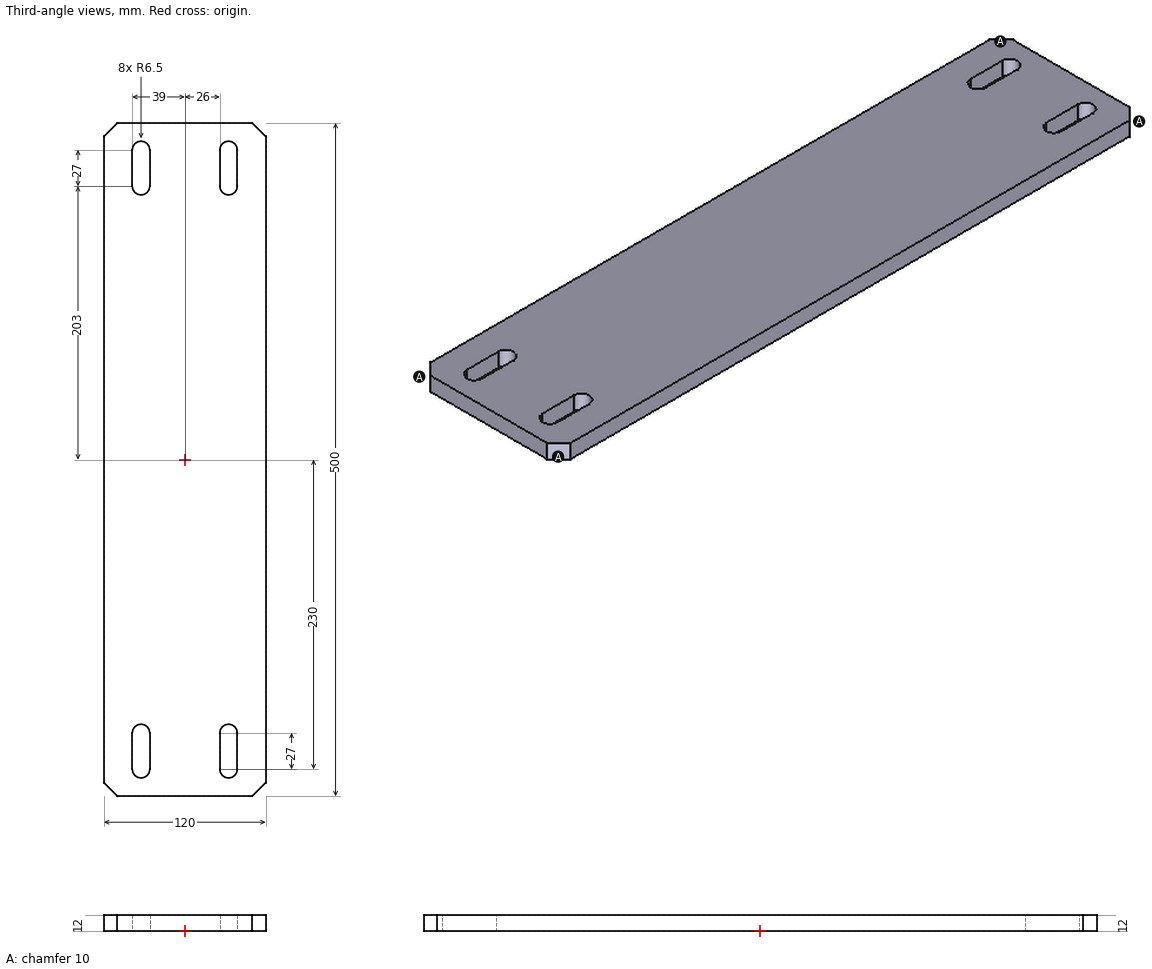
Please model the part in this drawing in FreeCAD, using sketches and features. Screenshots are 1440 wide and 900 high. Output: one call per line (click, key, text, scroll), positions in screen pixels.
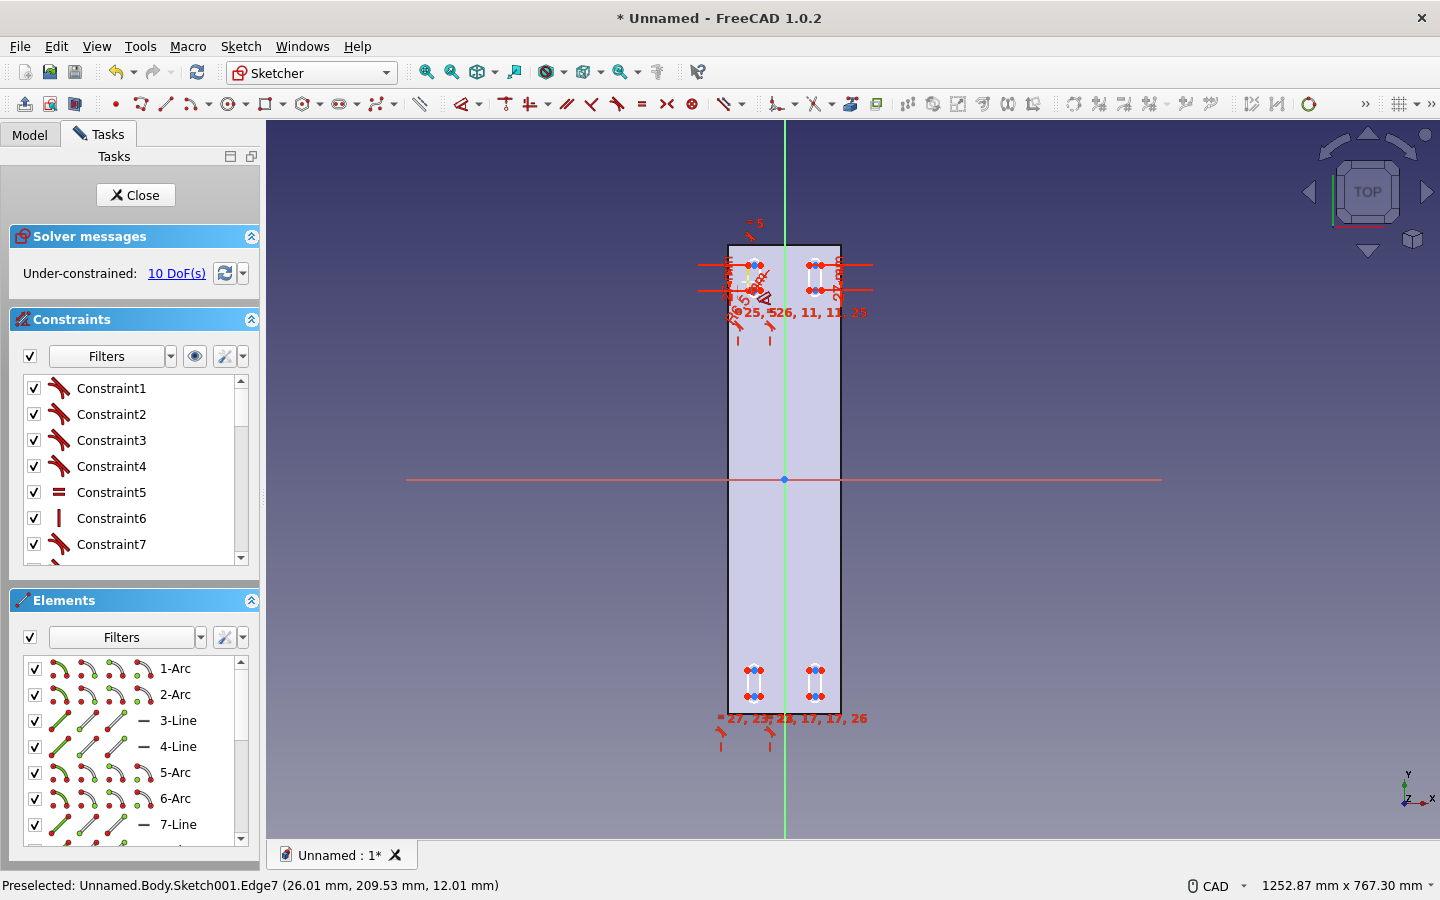
scroll(809, 689, up, 3)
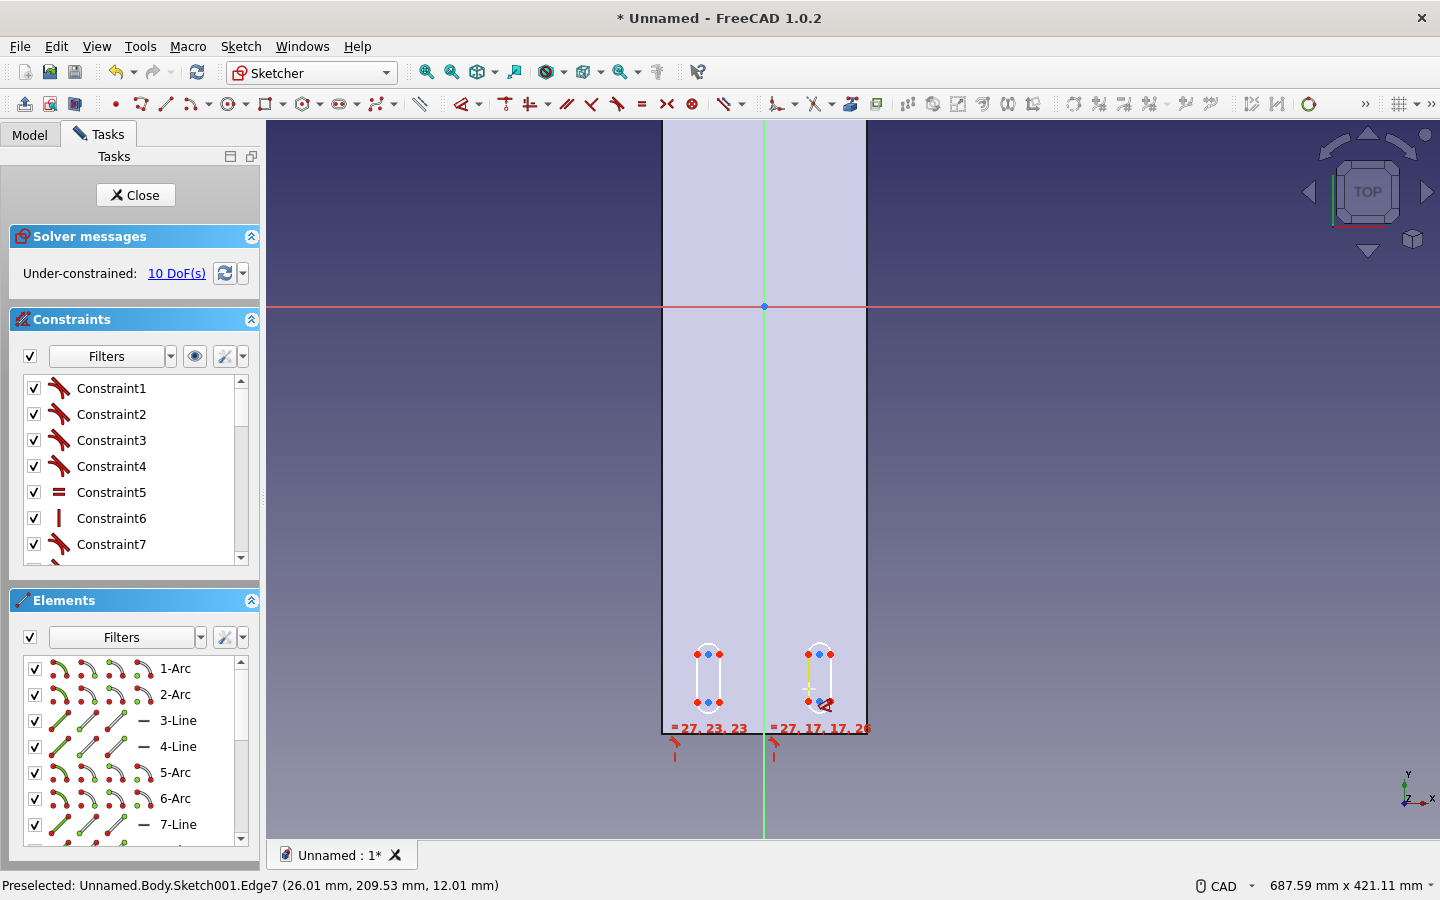
click(809, 687)
click(867, 678)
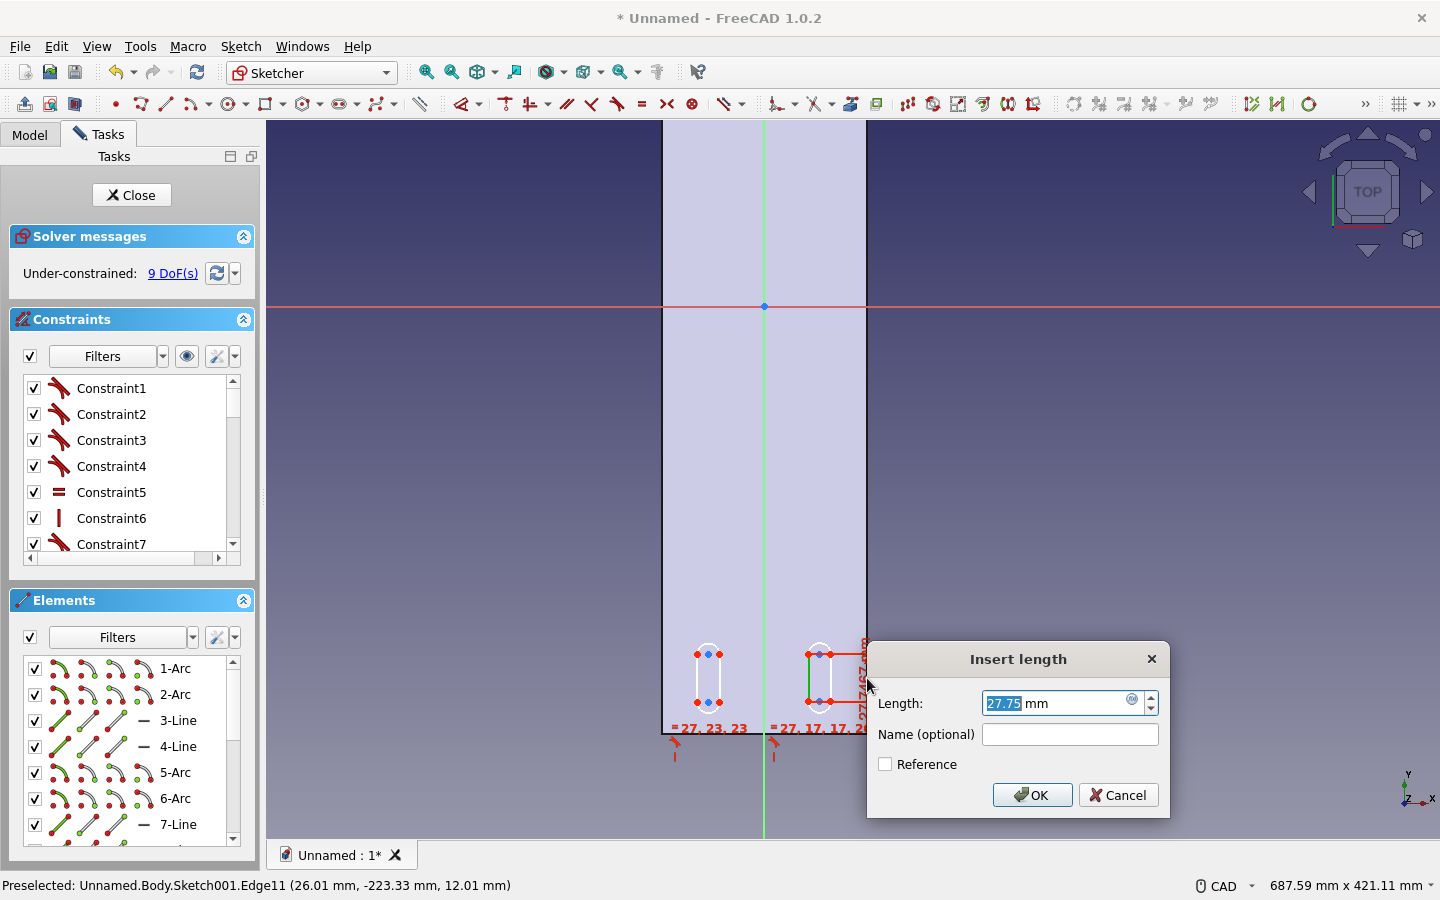
text(27)
key(Return)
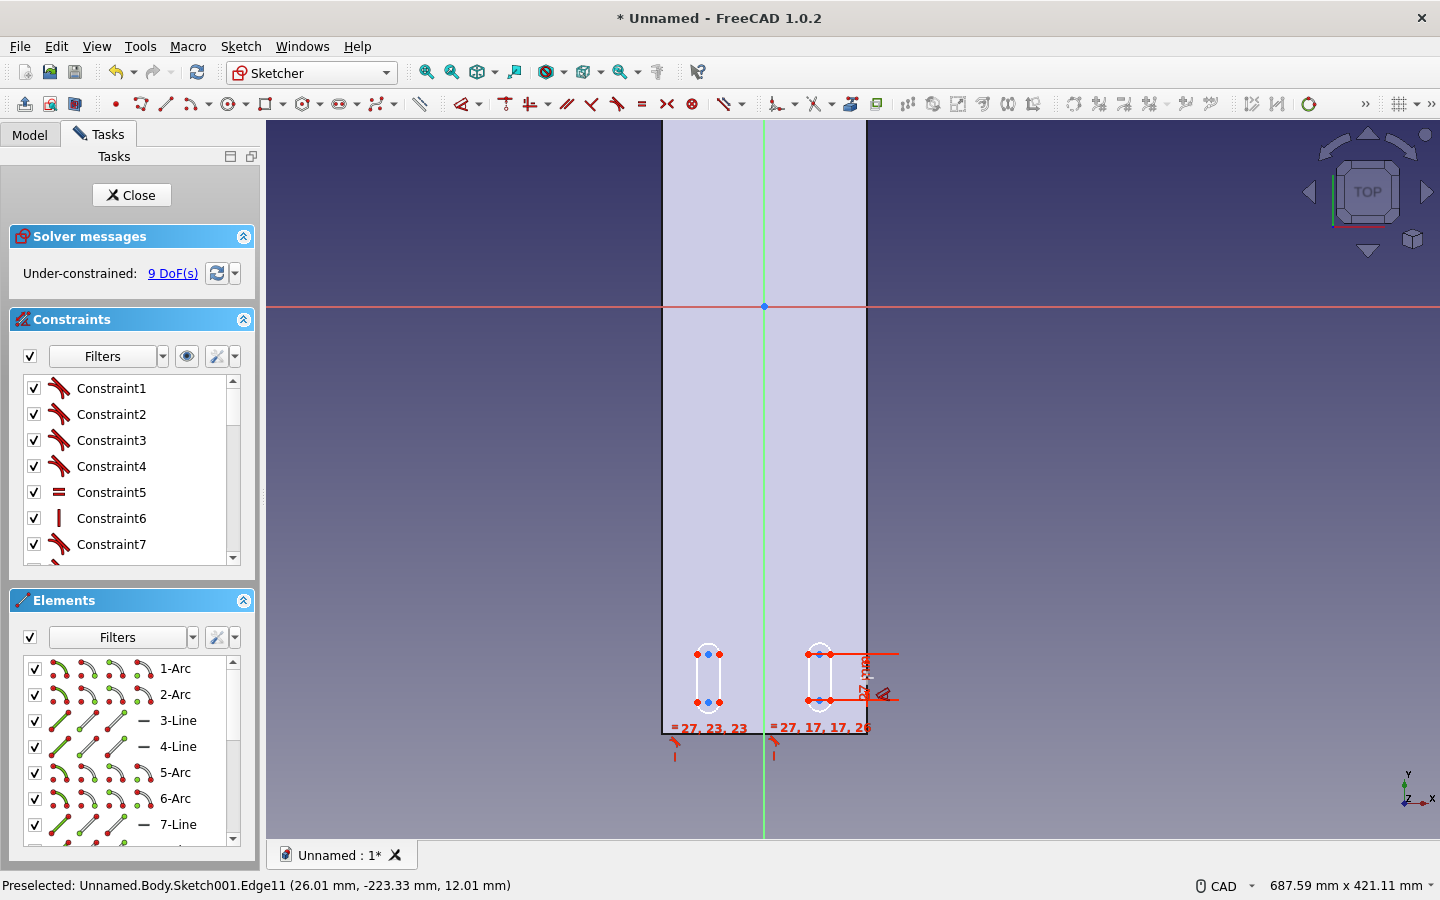
click(697, 688)
click(663, 678)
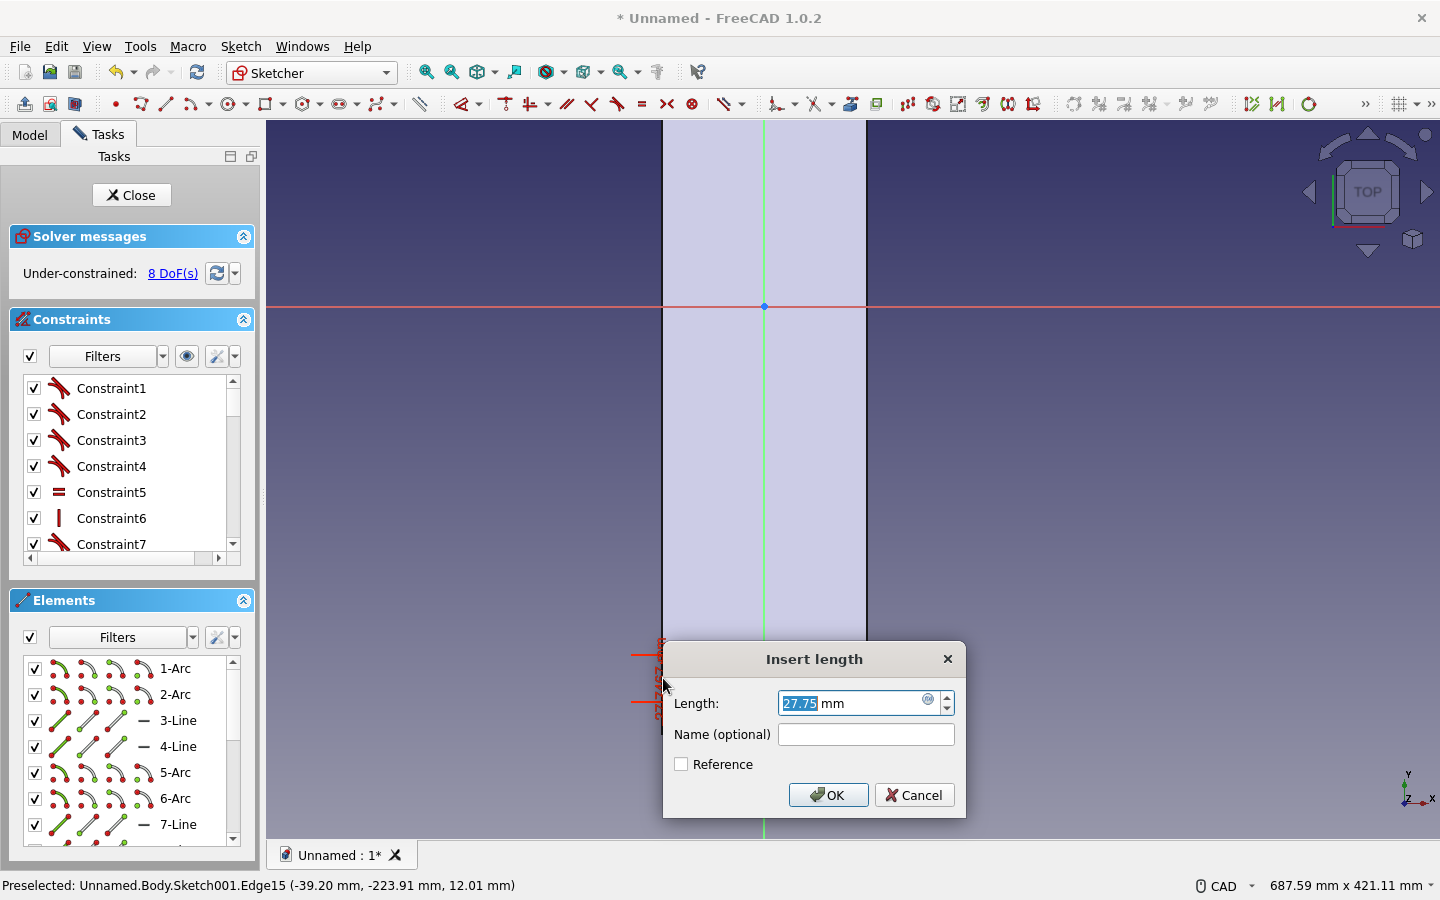
text(27)
key(Return)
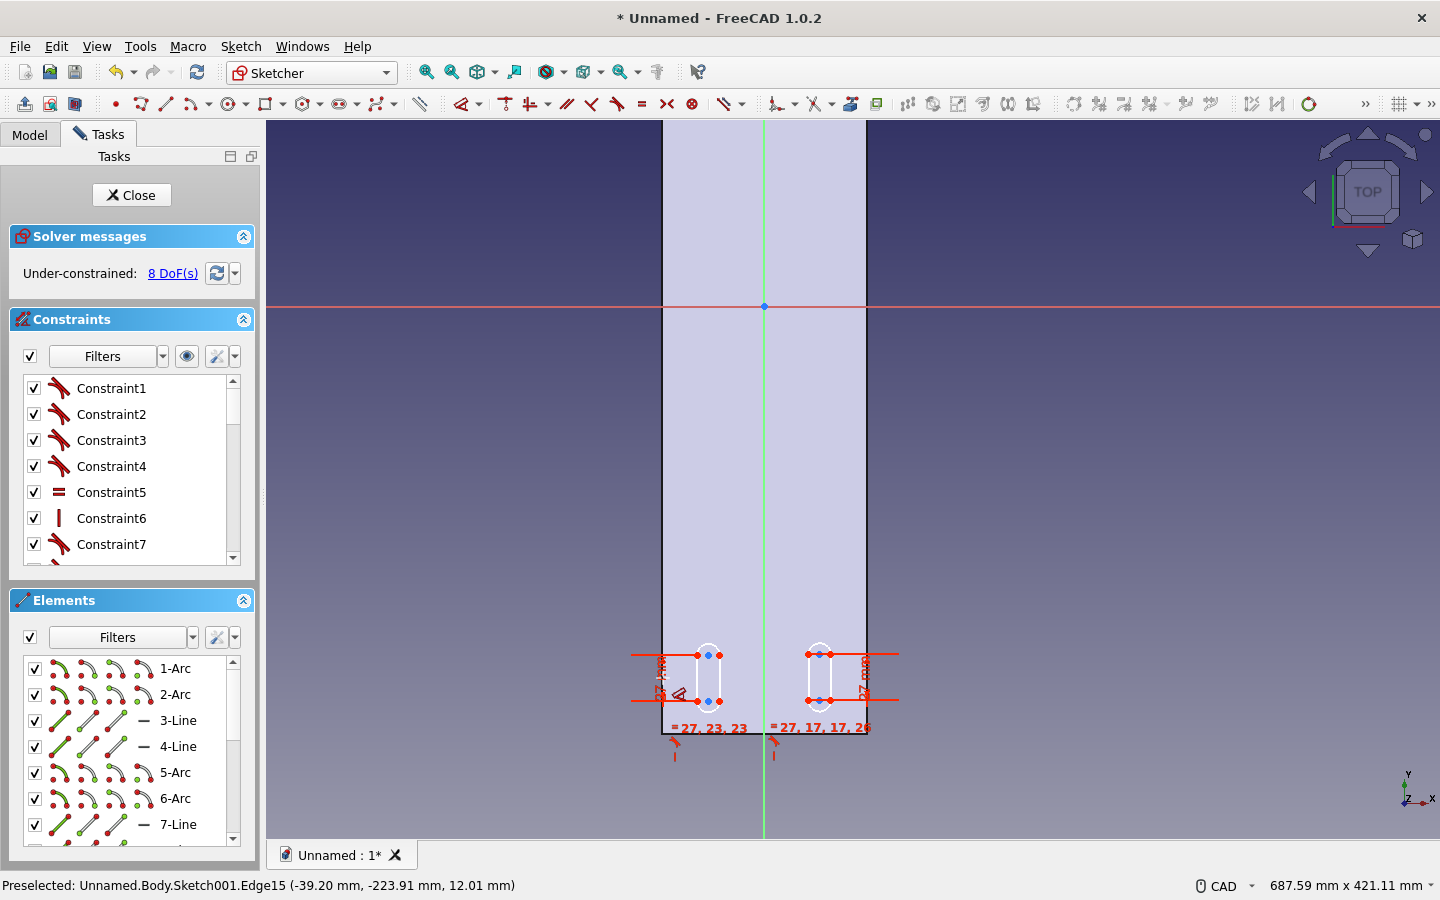
scroll(809, 690, down, 3)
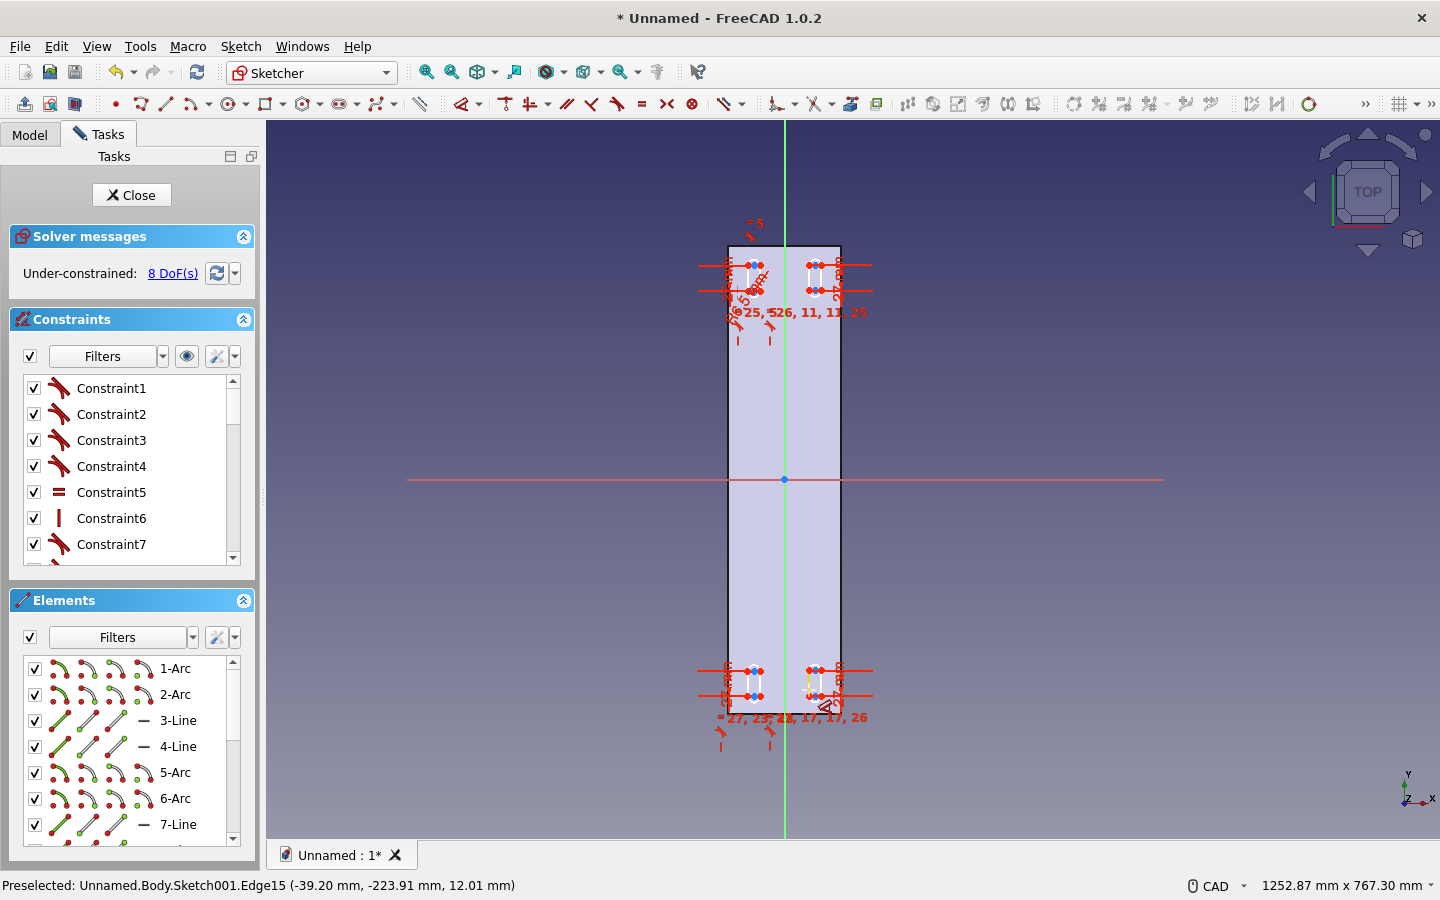
scroll(748, 291, up, 4)